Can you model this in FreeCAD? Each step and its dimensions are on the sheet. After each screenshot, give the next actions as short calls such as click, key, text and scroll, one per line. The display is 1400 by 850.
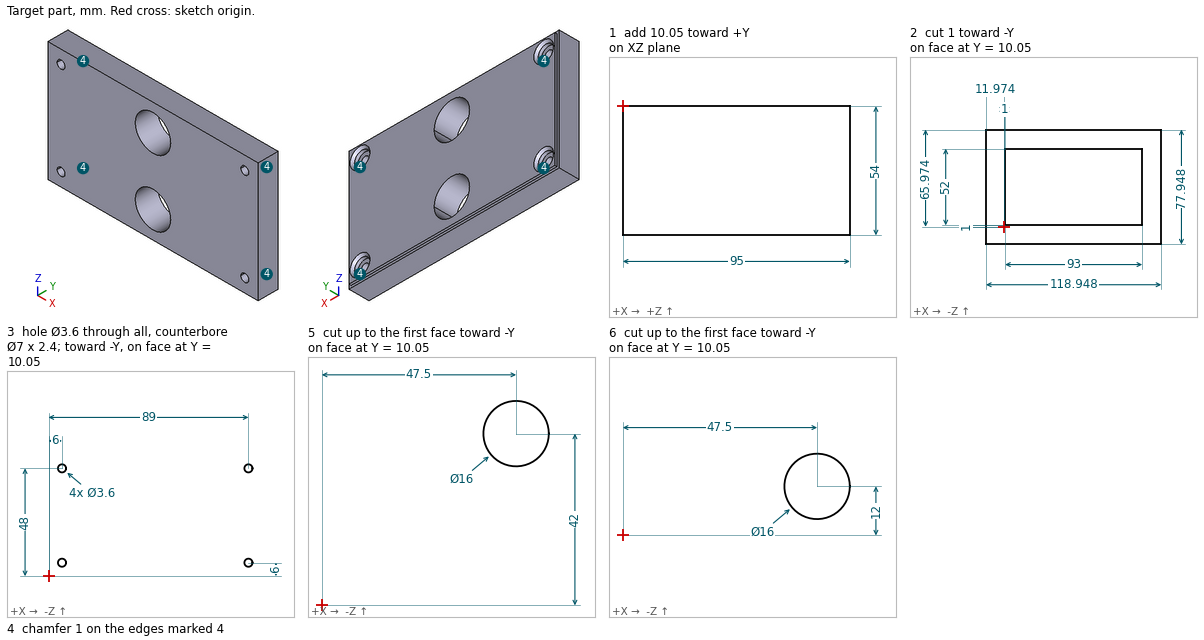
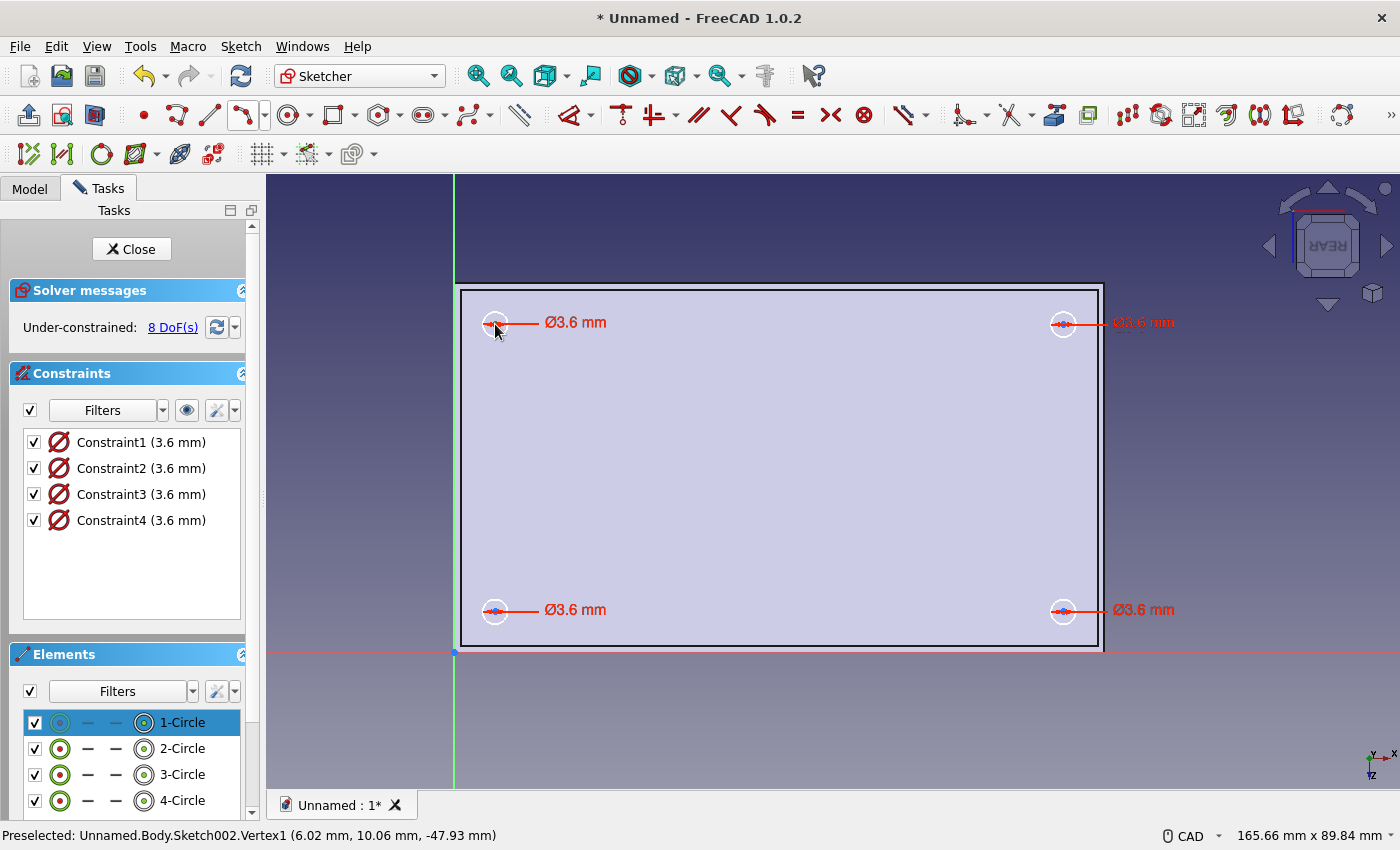
click(1063, 325)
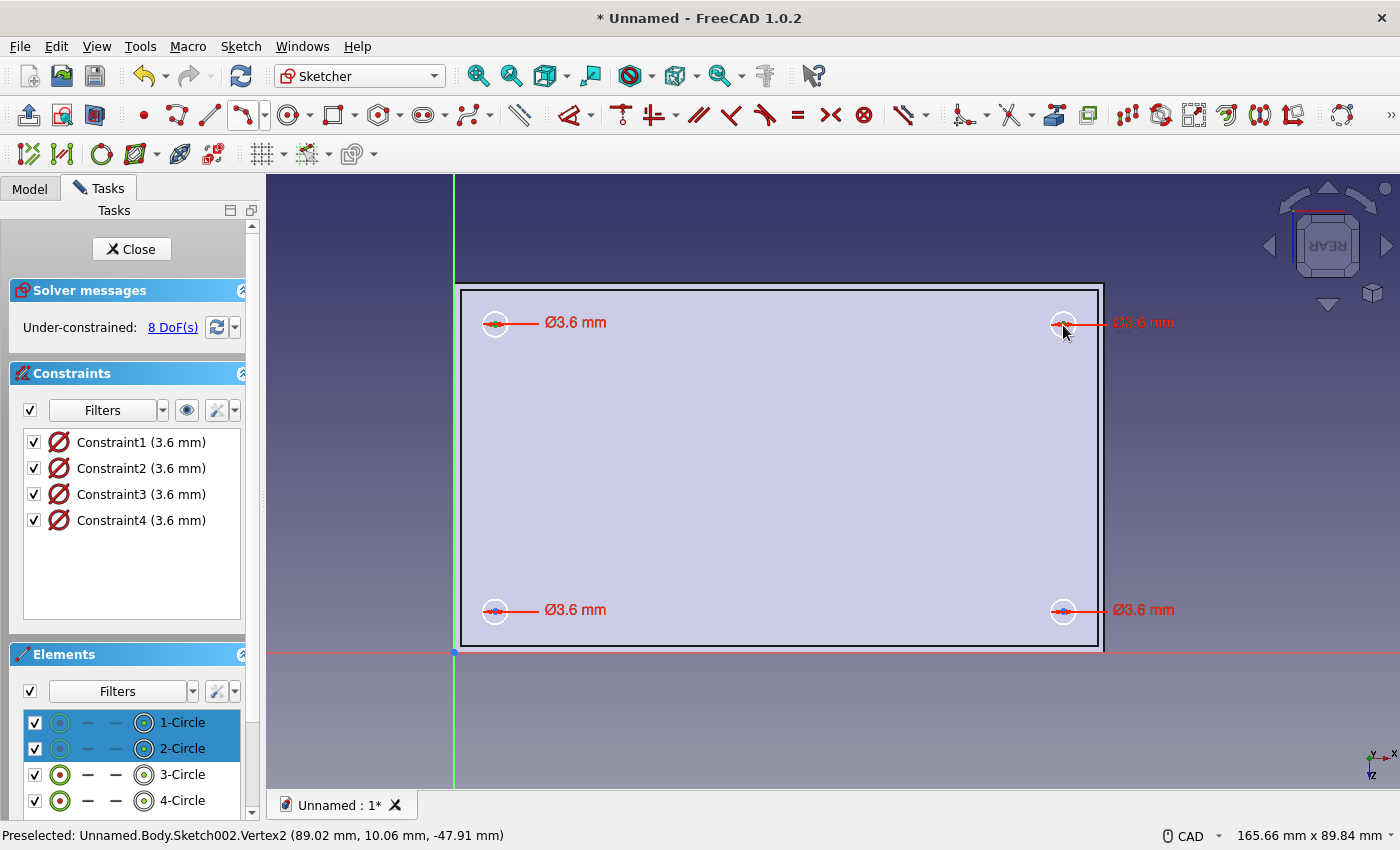
click(676, 116)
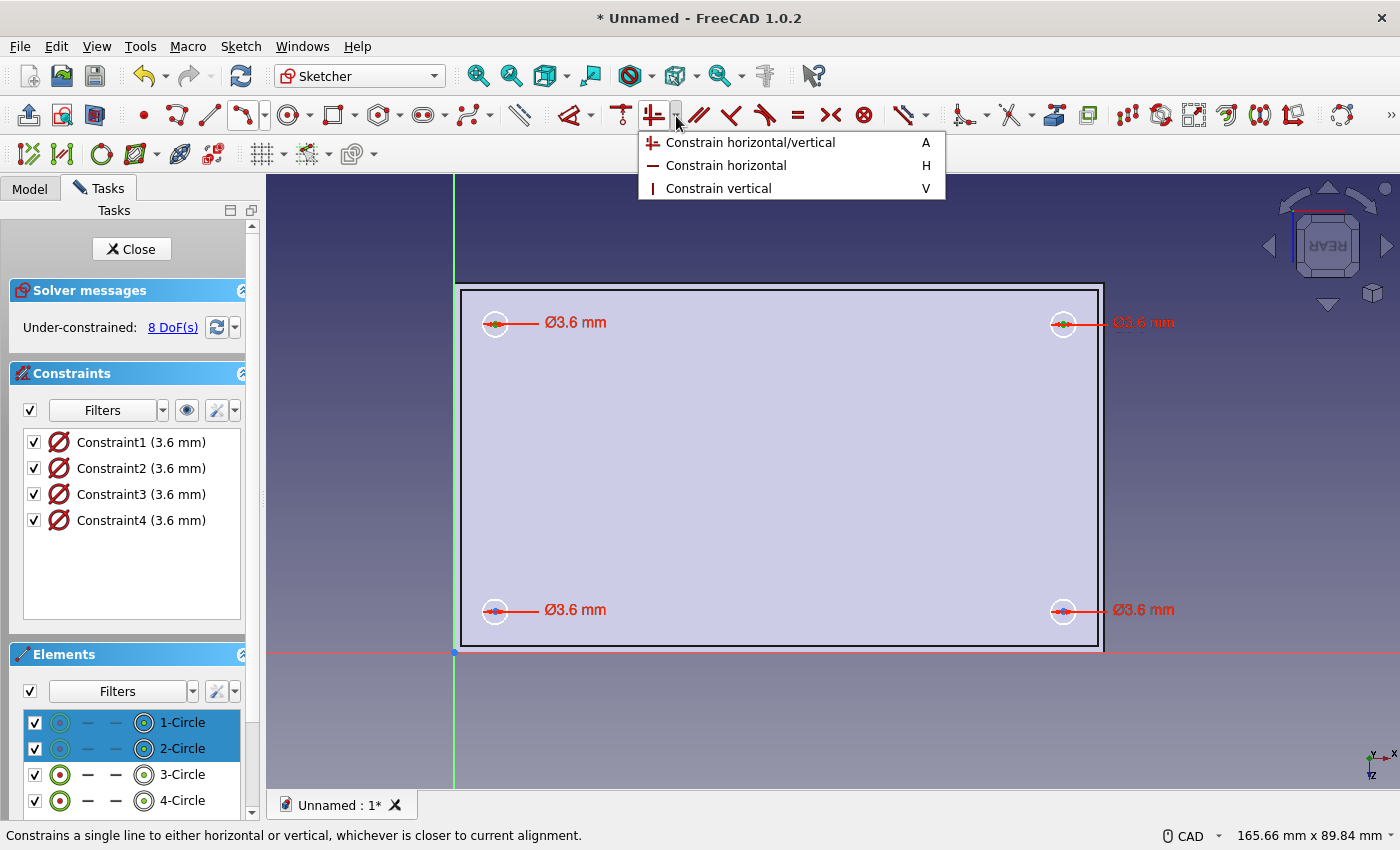
click(792, 166)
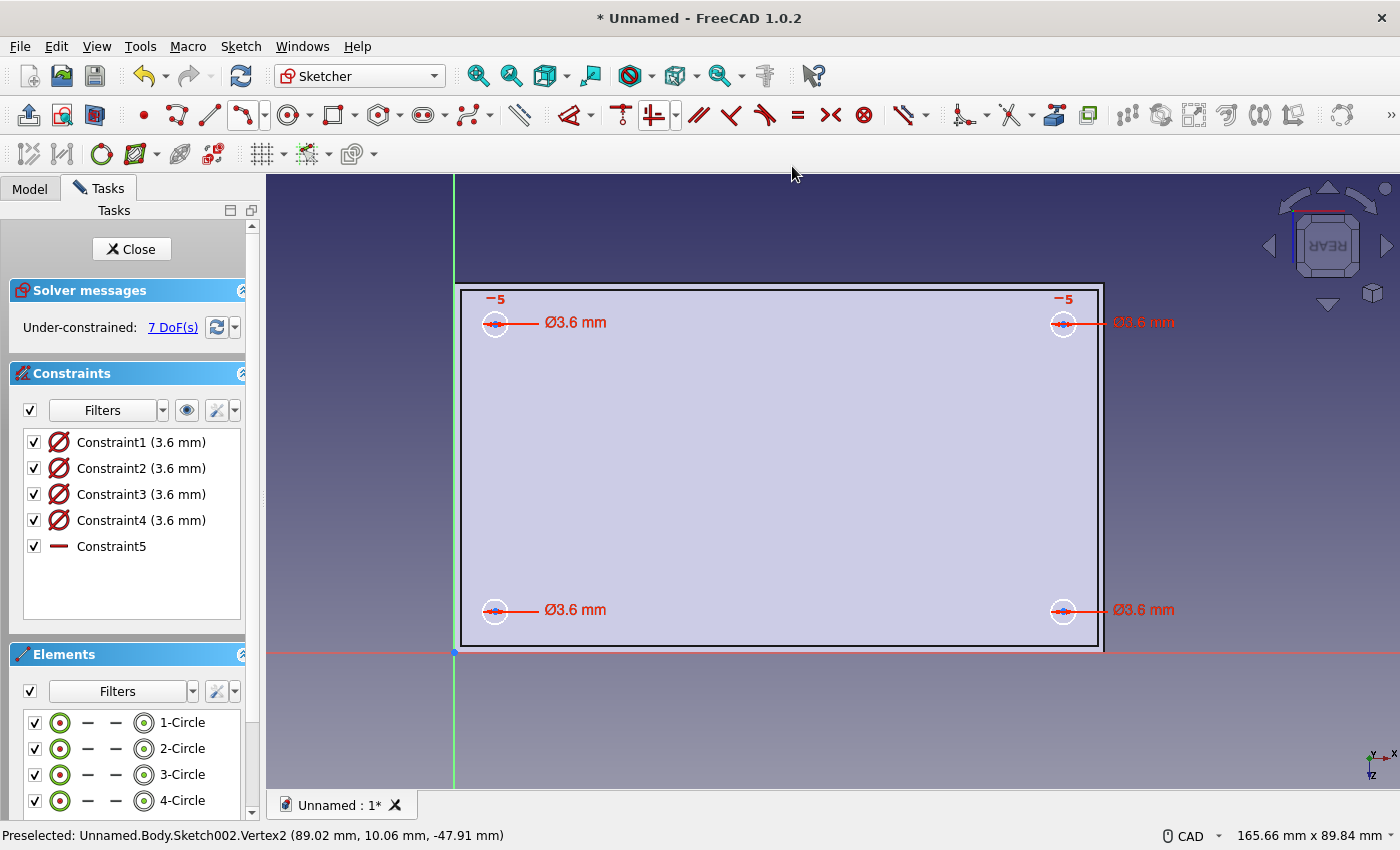
click(1063, 324)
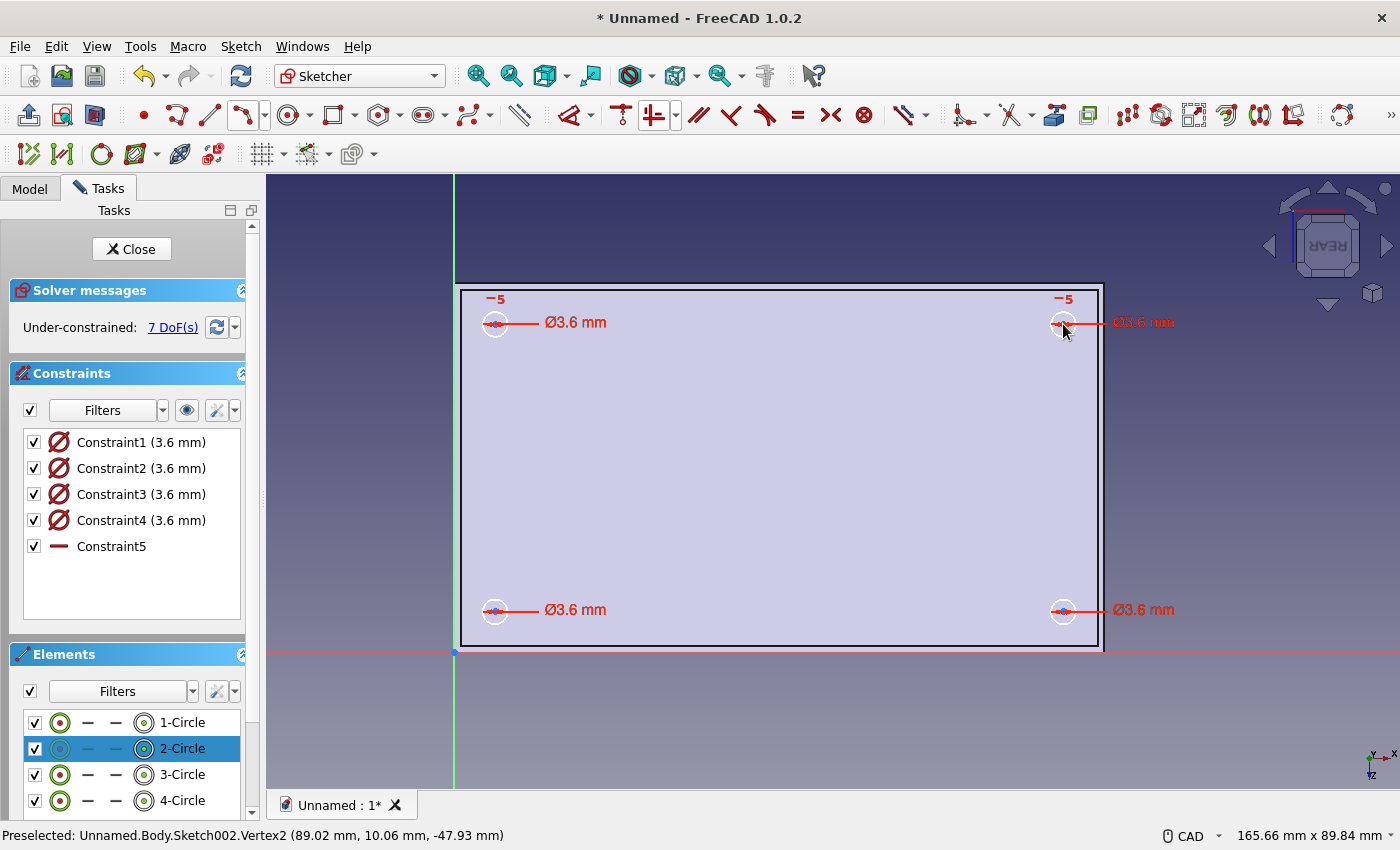
click(1063, 612)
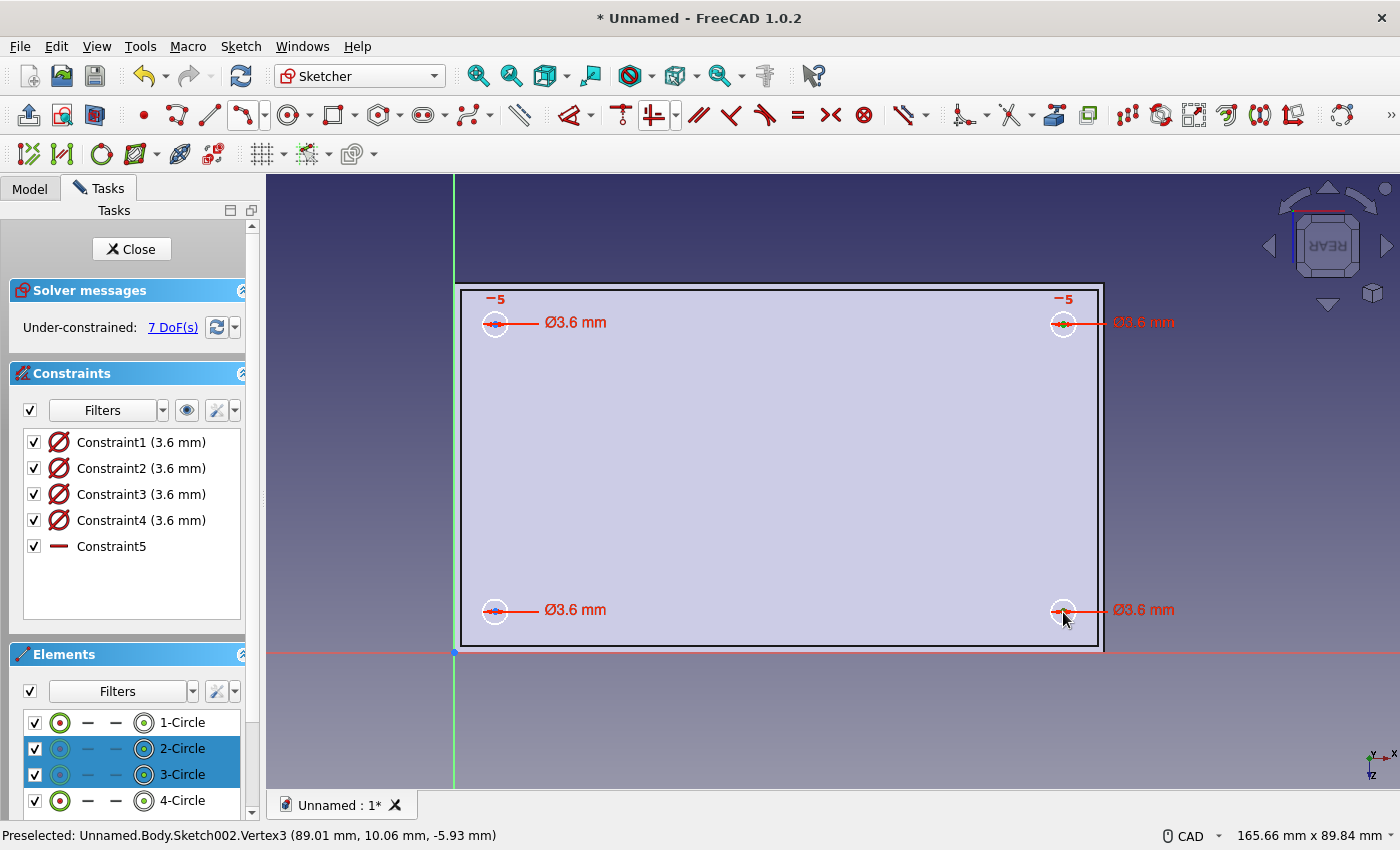
click(676, 116)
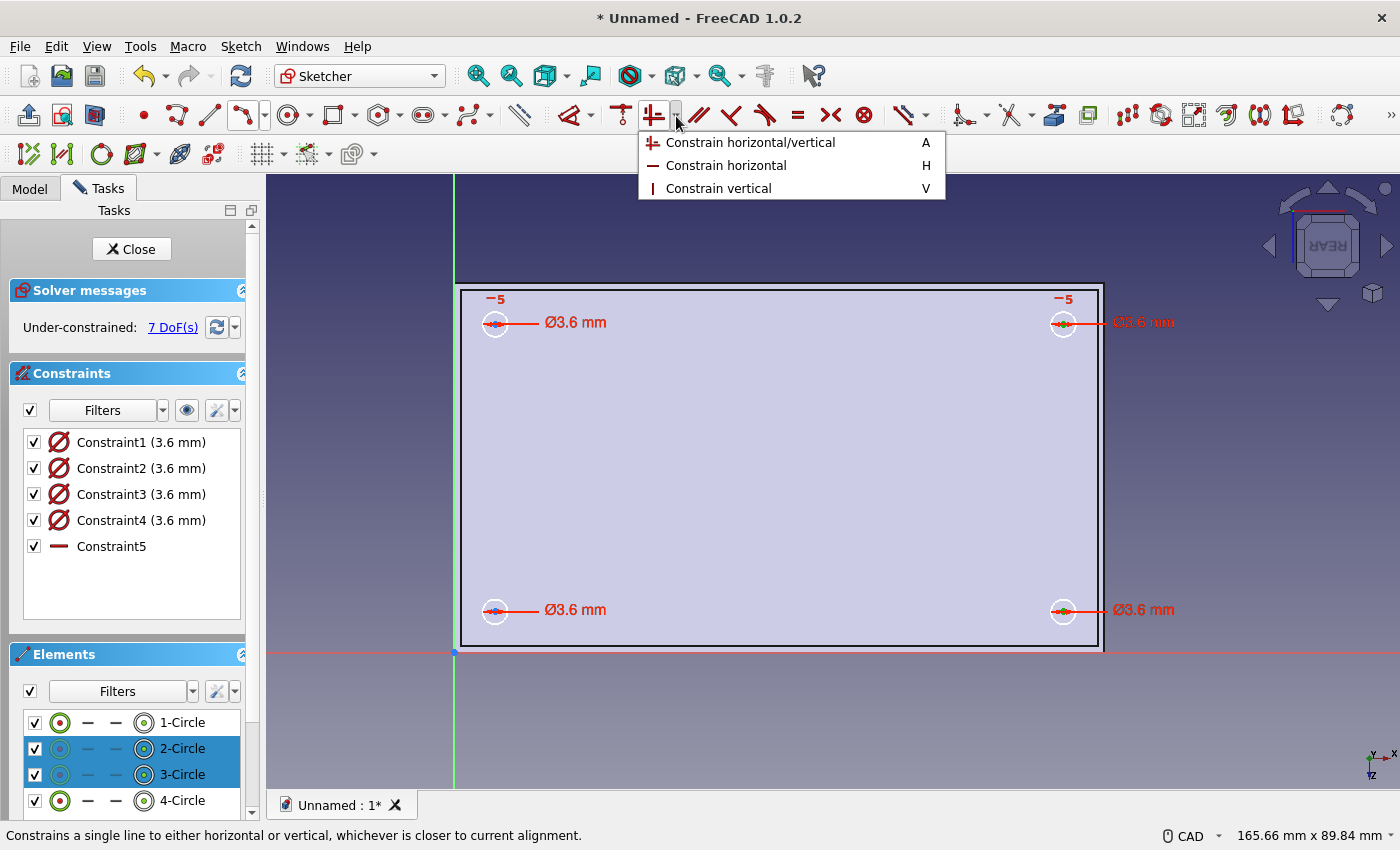
click(792, 188)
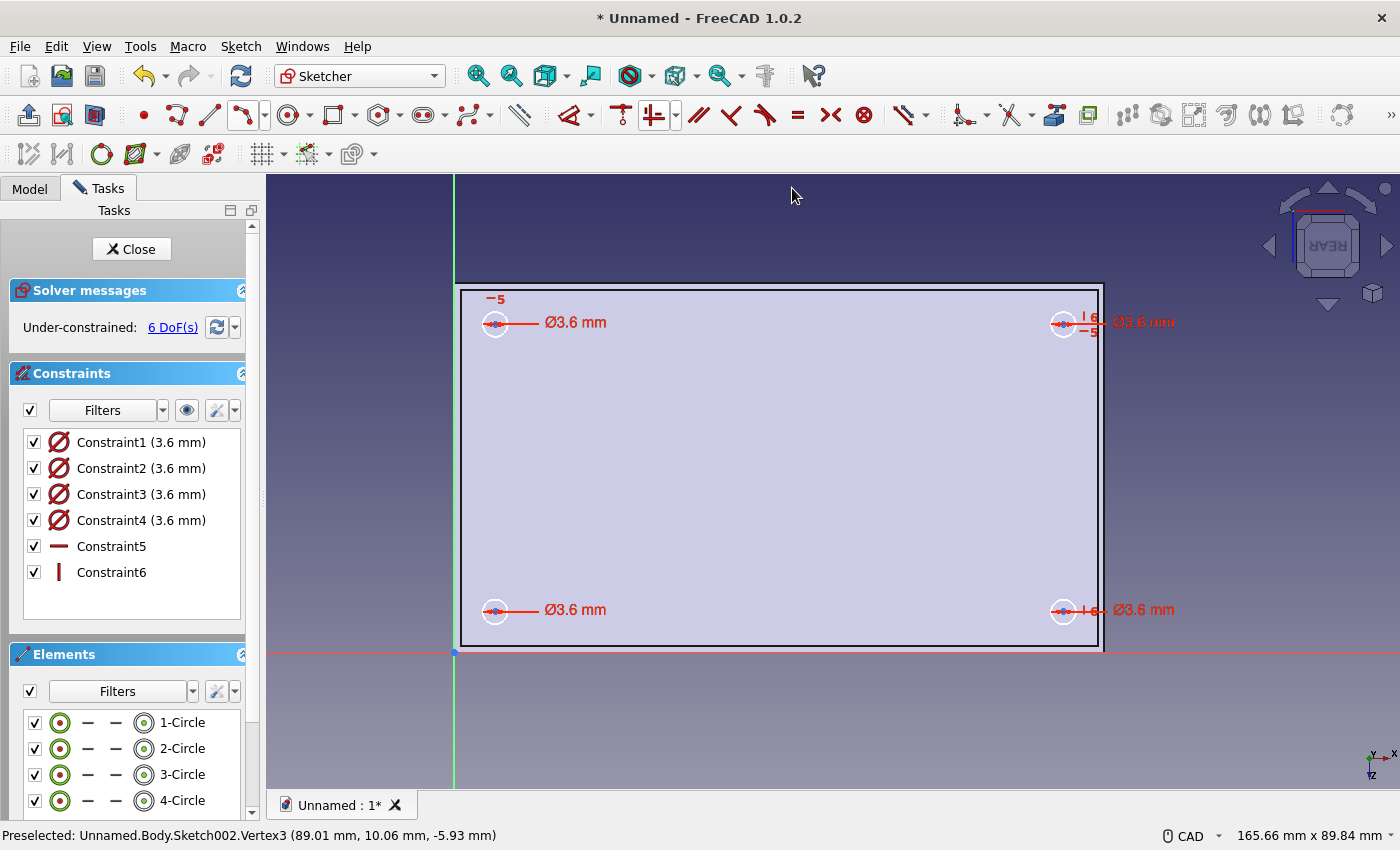
click(495, 324)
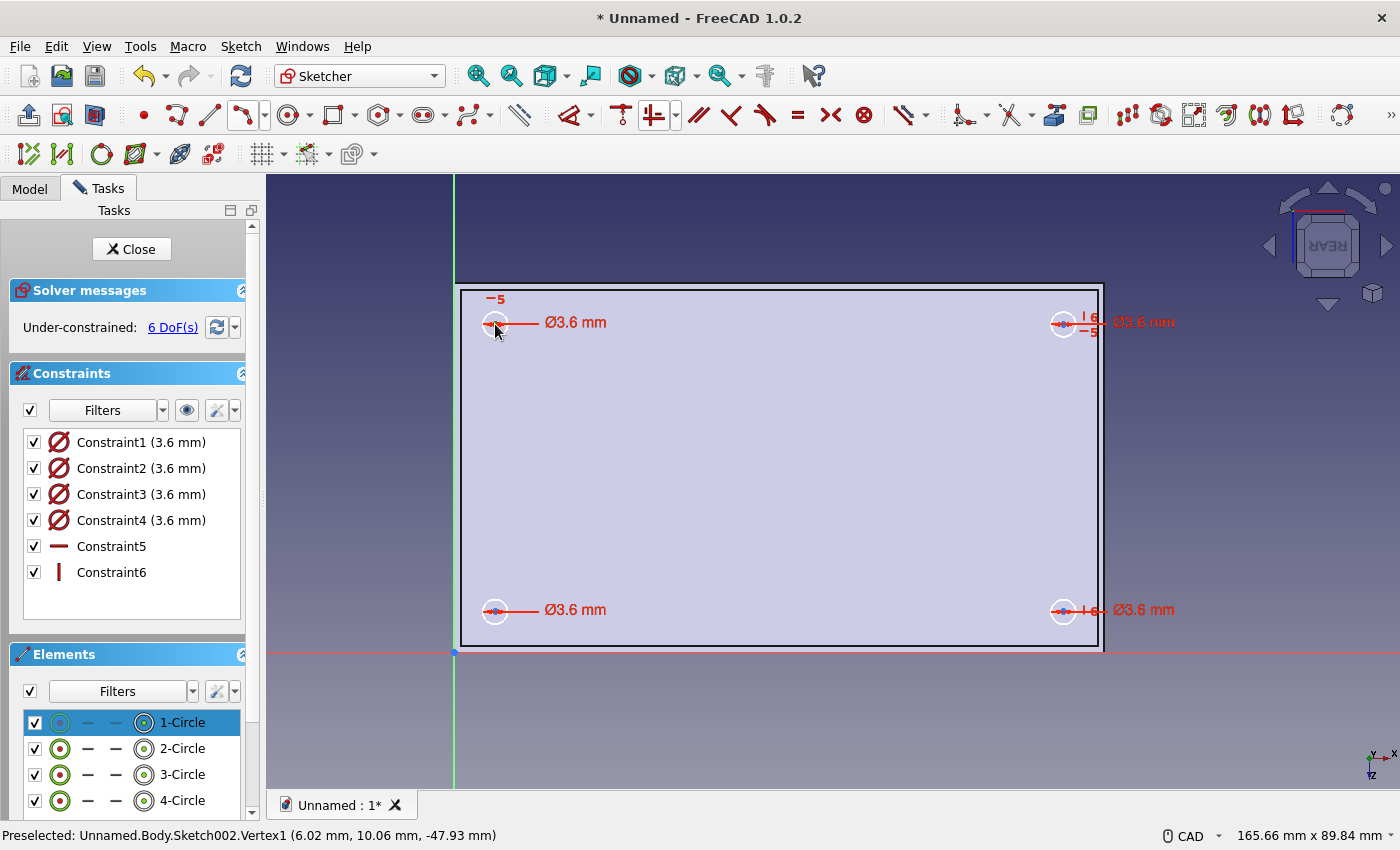
click(495, 612)